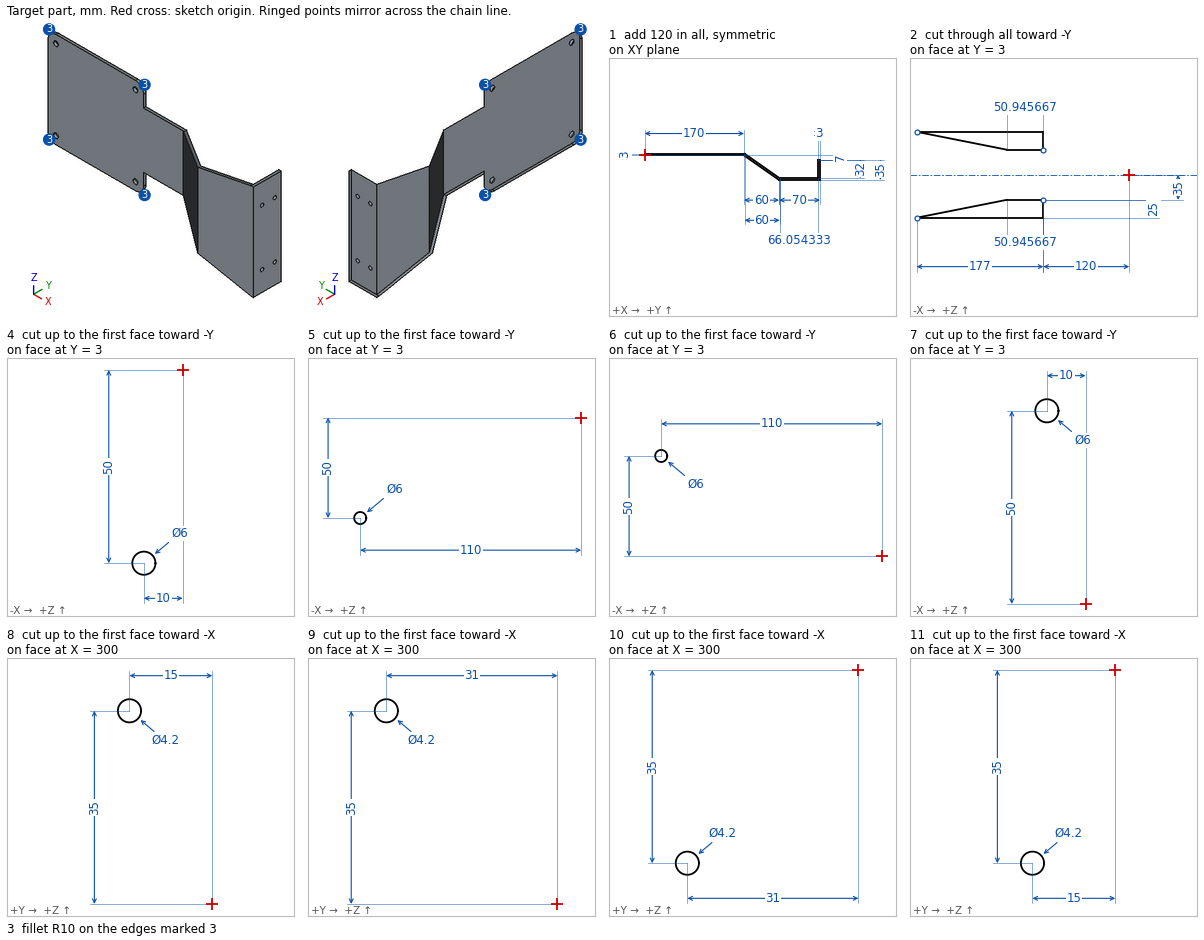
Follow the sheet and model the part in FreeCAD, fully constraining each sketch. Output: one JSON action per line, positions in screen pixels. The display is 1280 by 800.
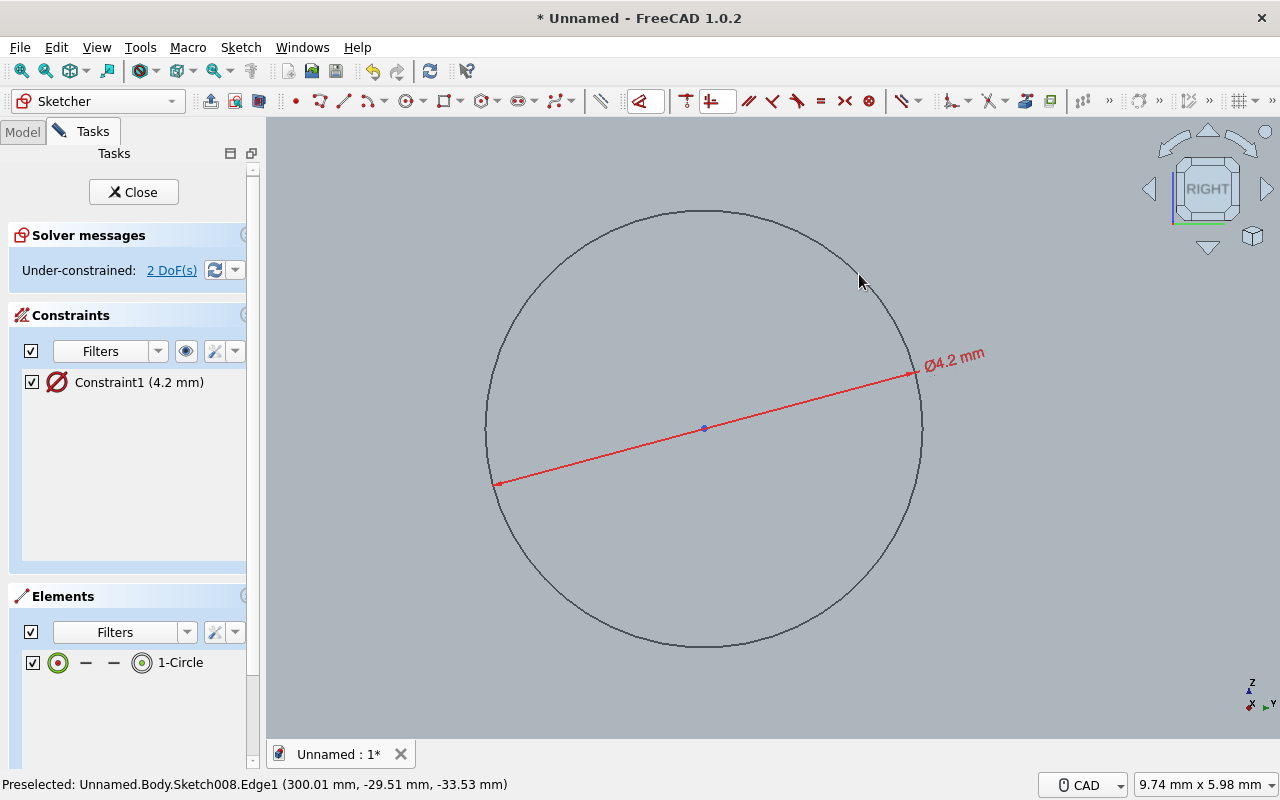
{"action": "left_click", "coordinate": [704, 429]}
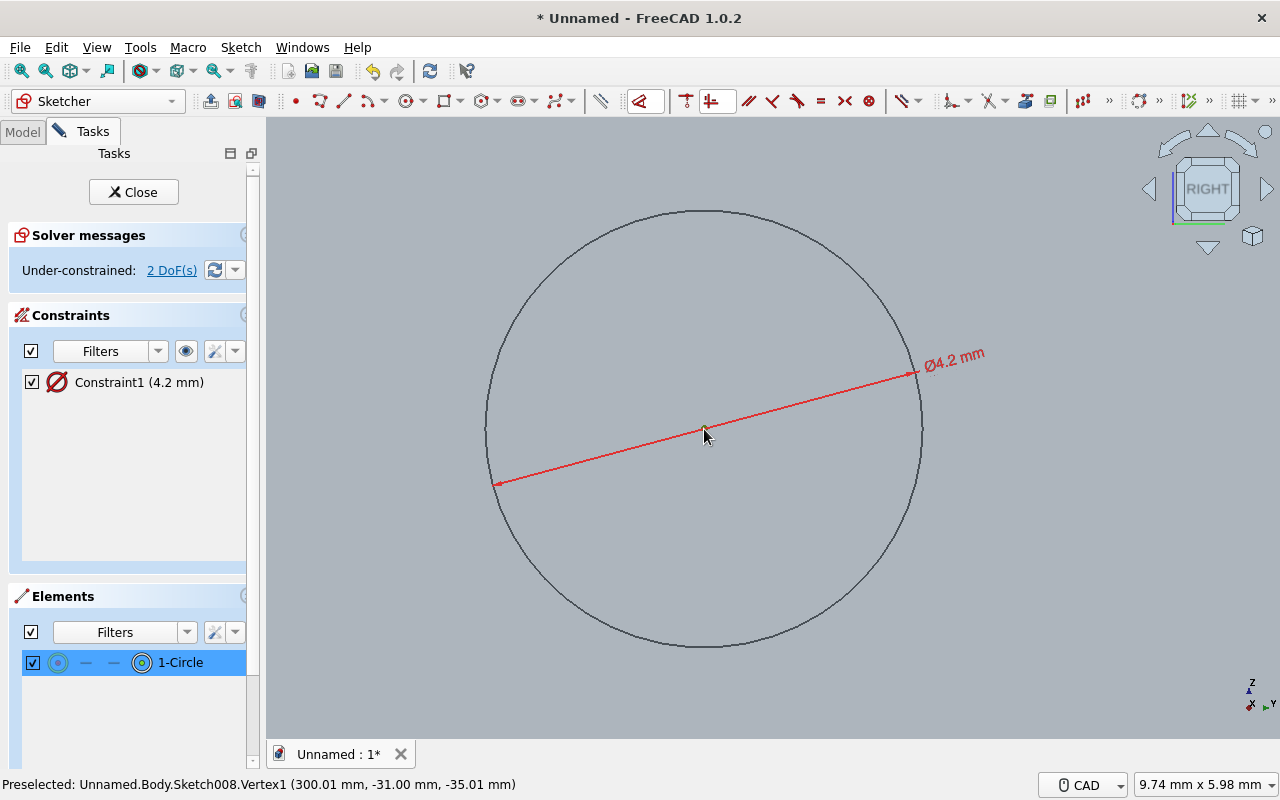
{"action": "key", "text": "l"}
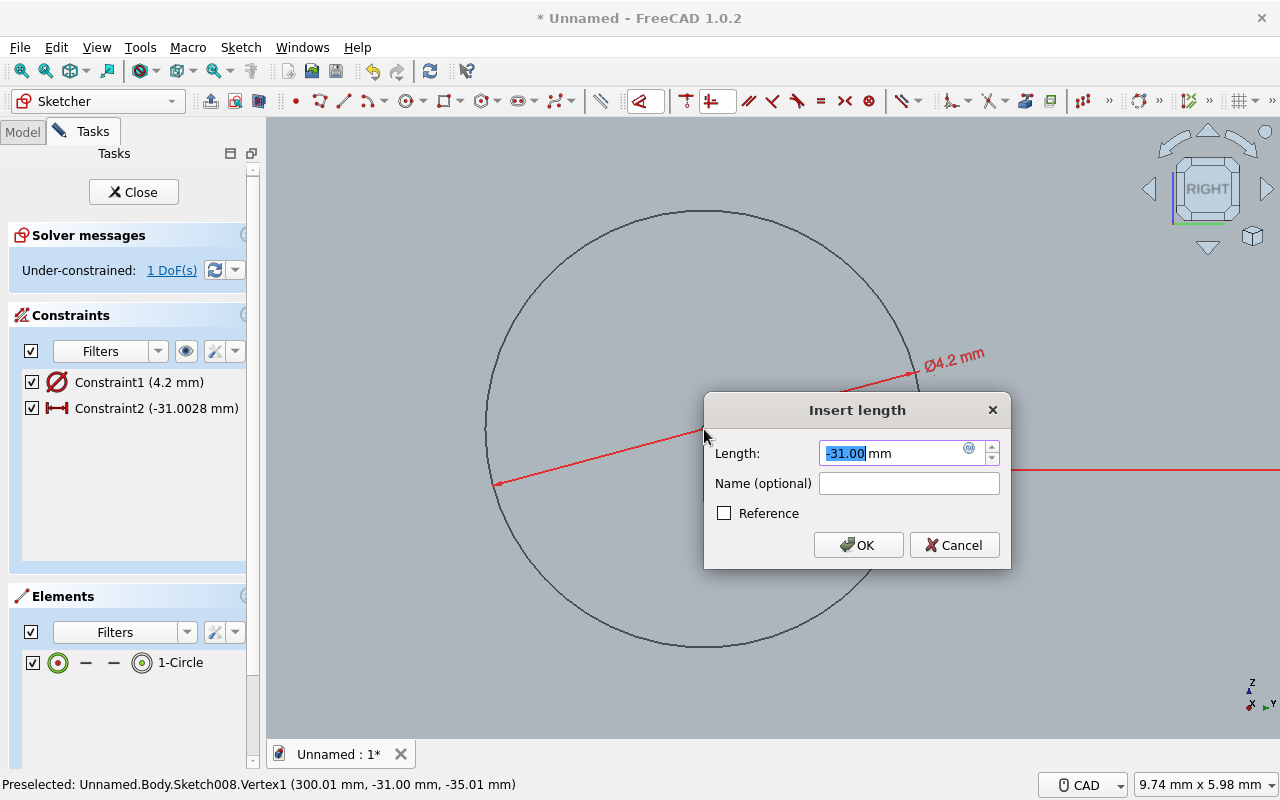
{"action": "type", "text": "-31"}
{"action": "key", "text": "Return"}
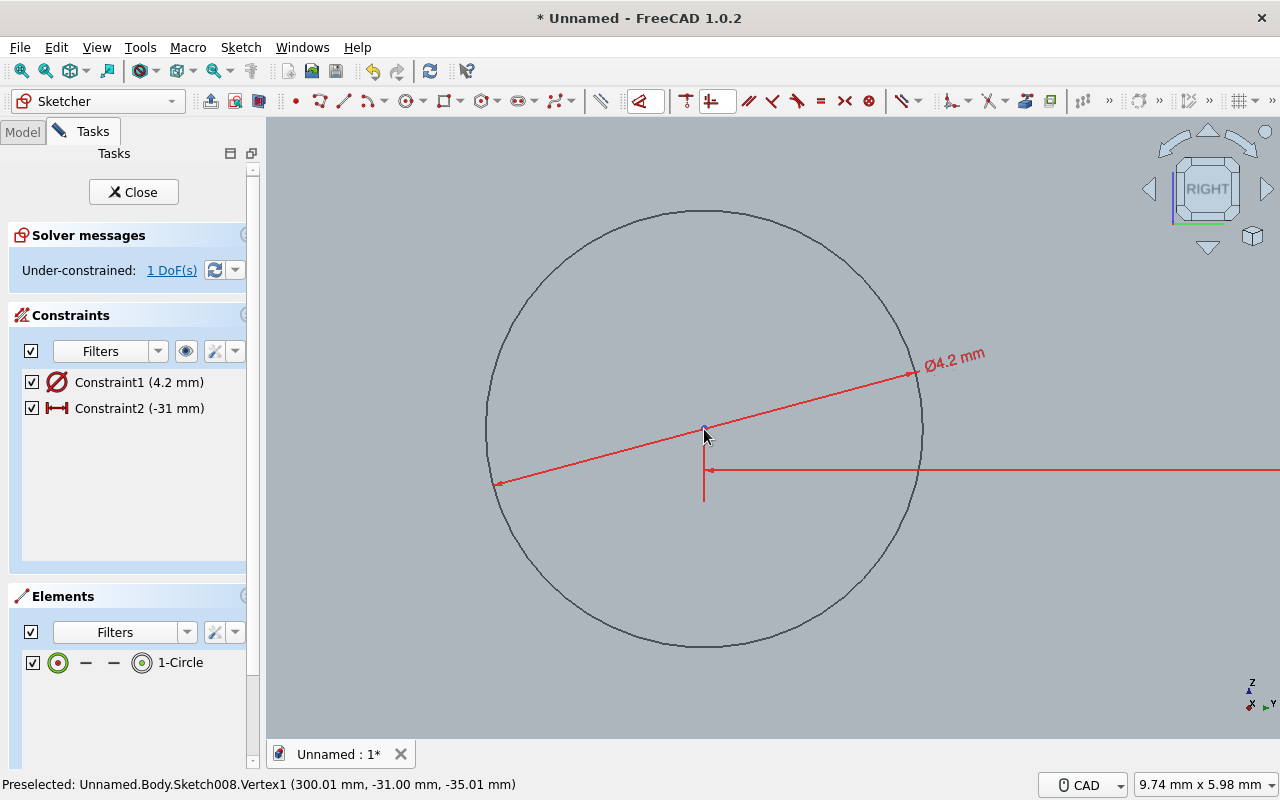
{"action": "left_click", "coordinate": [704, 429]}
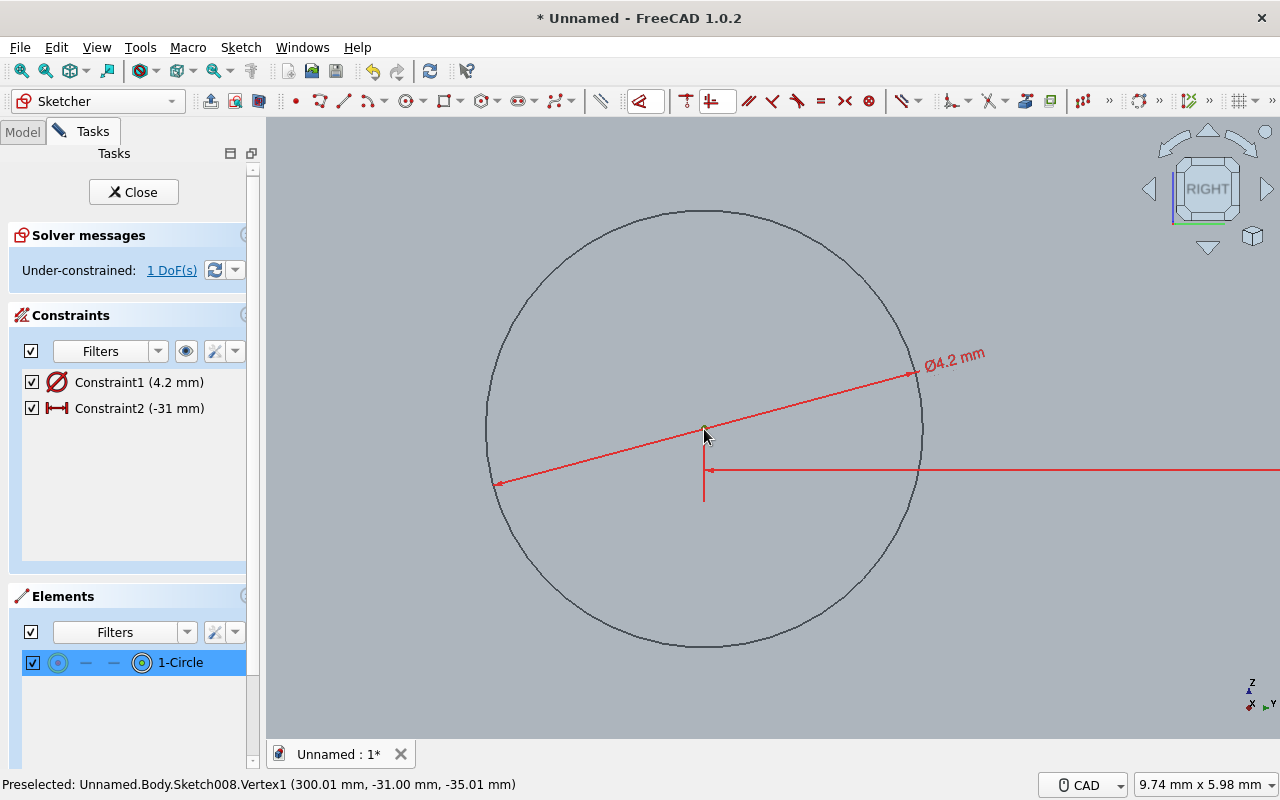
{"action": "key", "text": "i"}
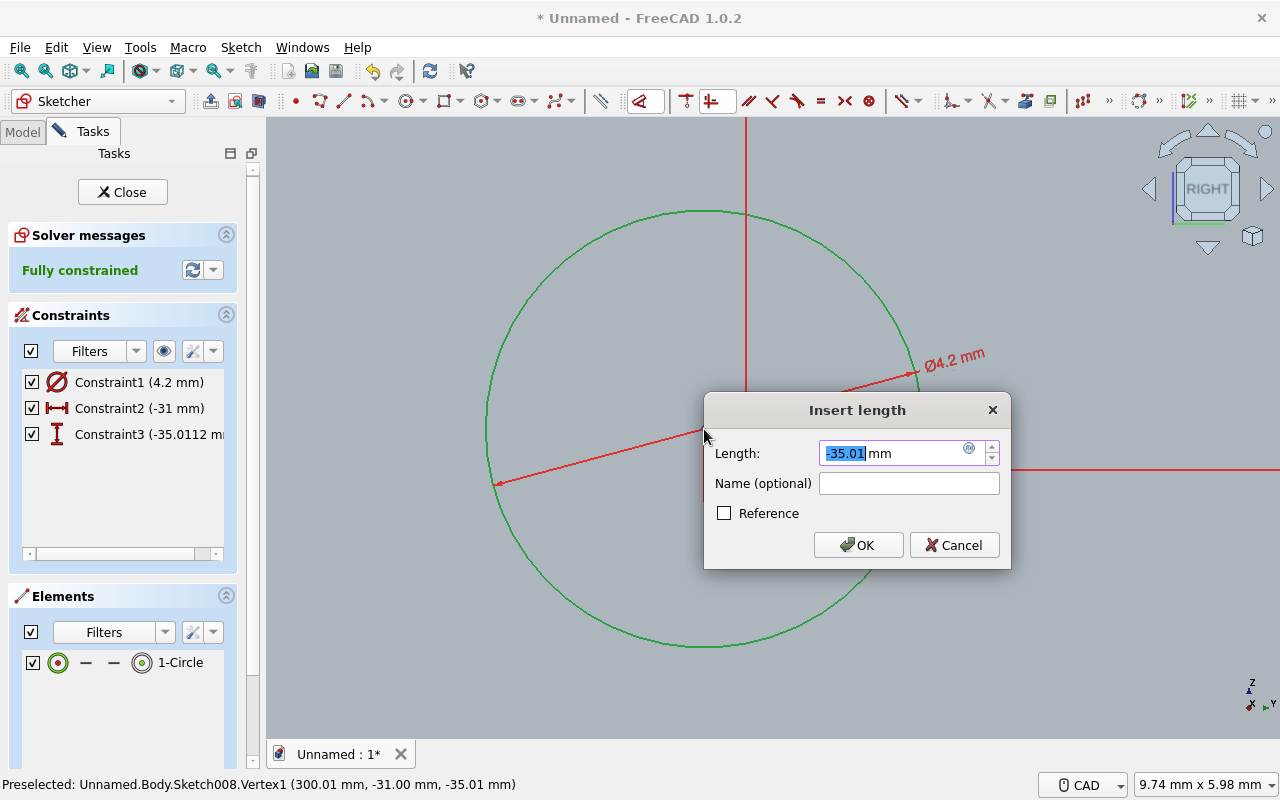
{"action": "type", "text": "-35"}
{"action": "key", "text": "Return"}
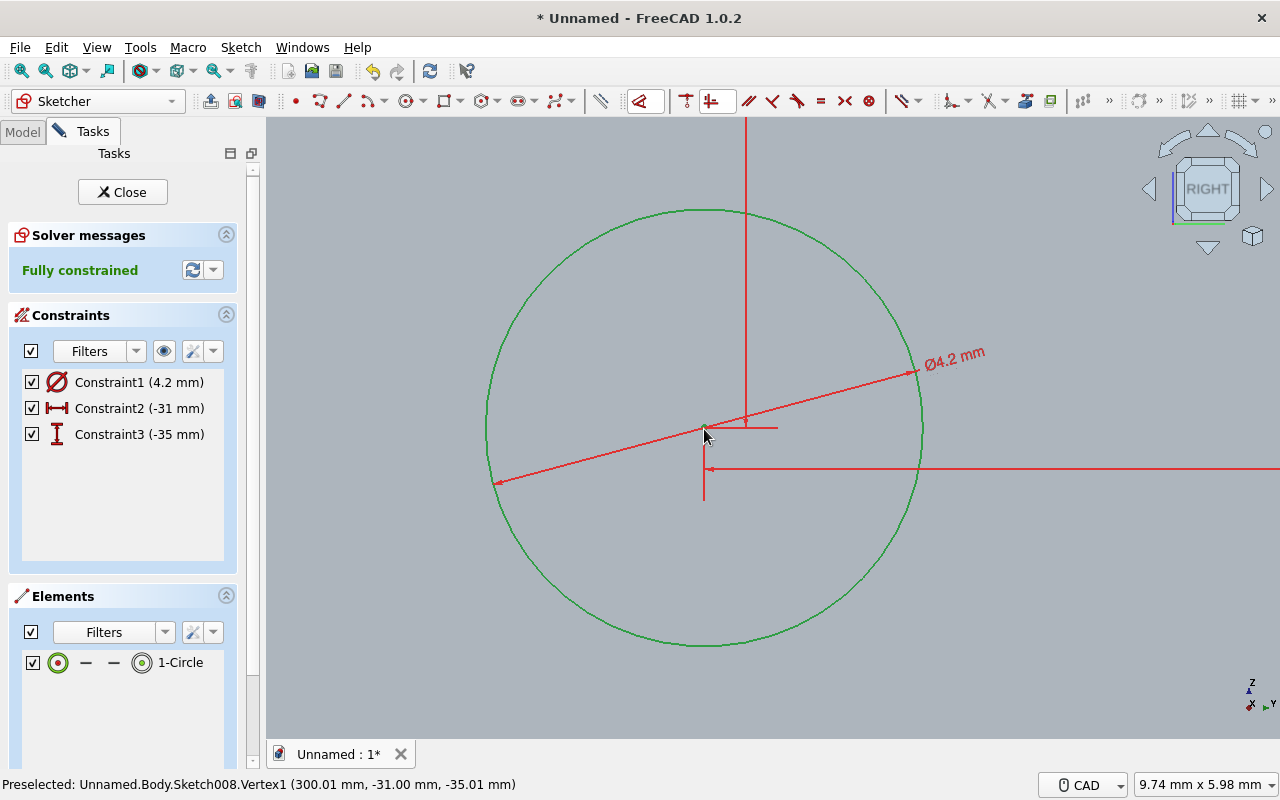
{"action": "left_click", "coordinate": [123, 192]}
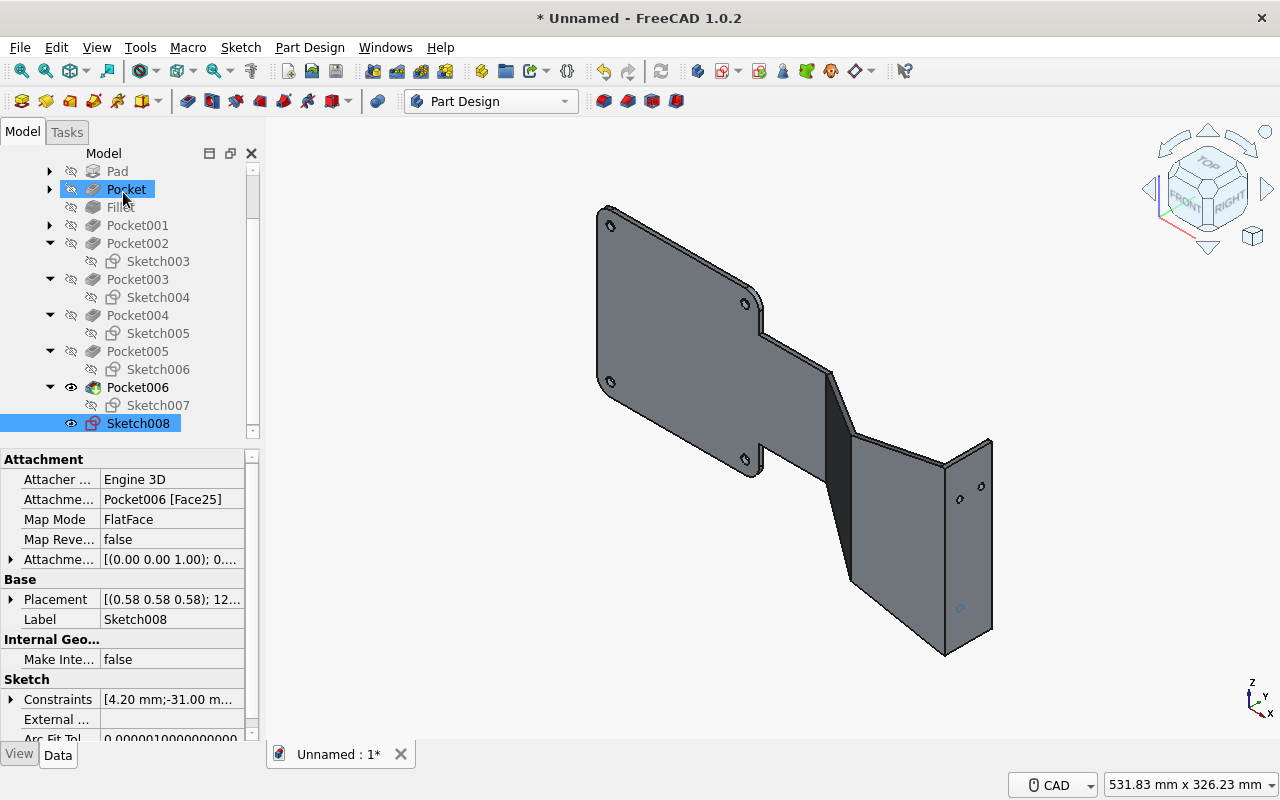
{"action": "left_click", "coordinate": [188, 102]}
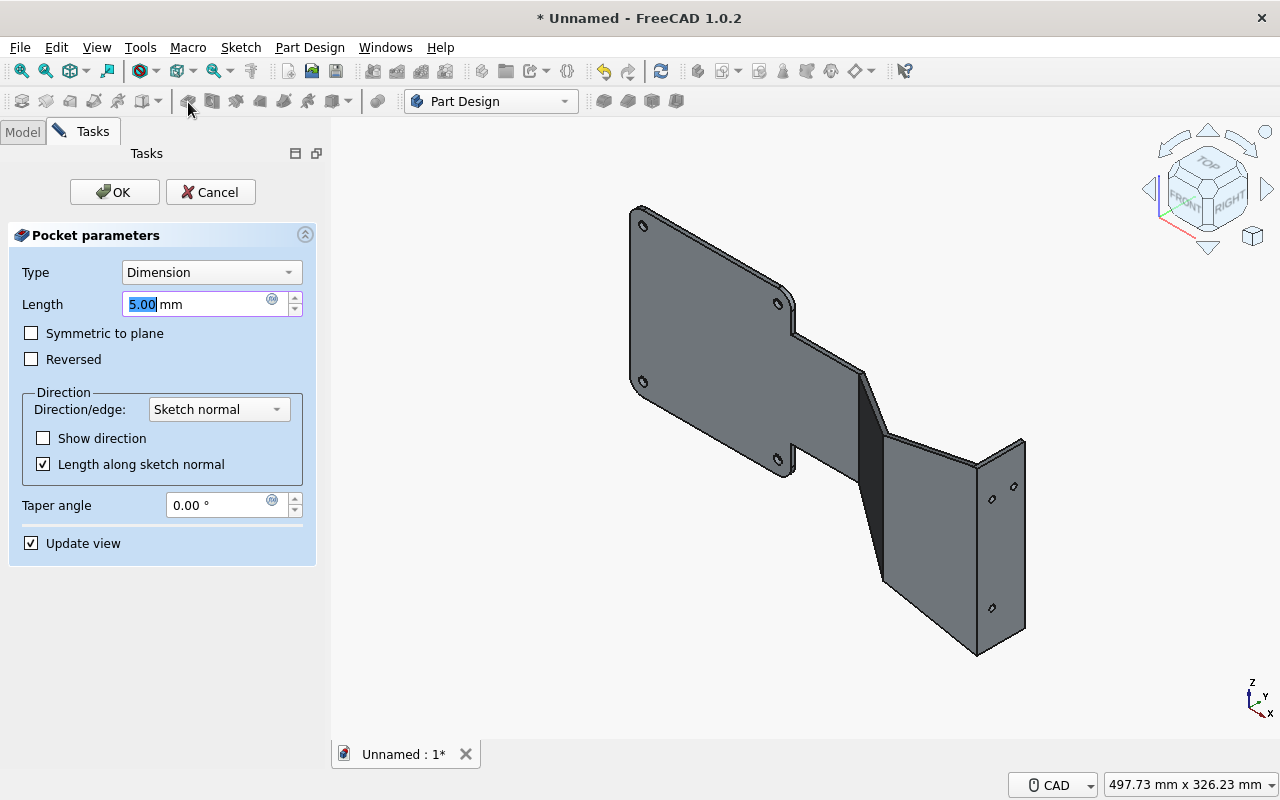
{"action": "left_click", "coordinate": [212, 272]}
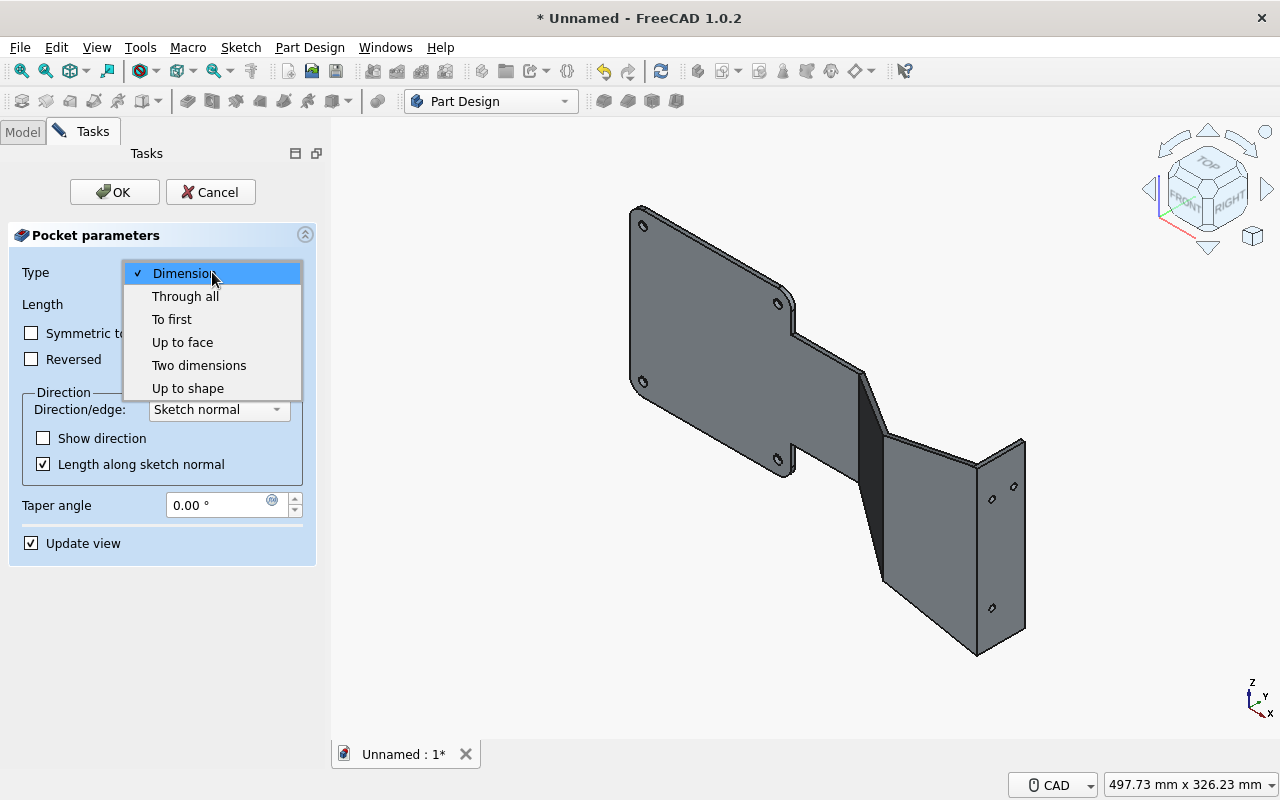
{"action": "left_click", "coordinate": [212, 320]}